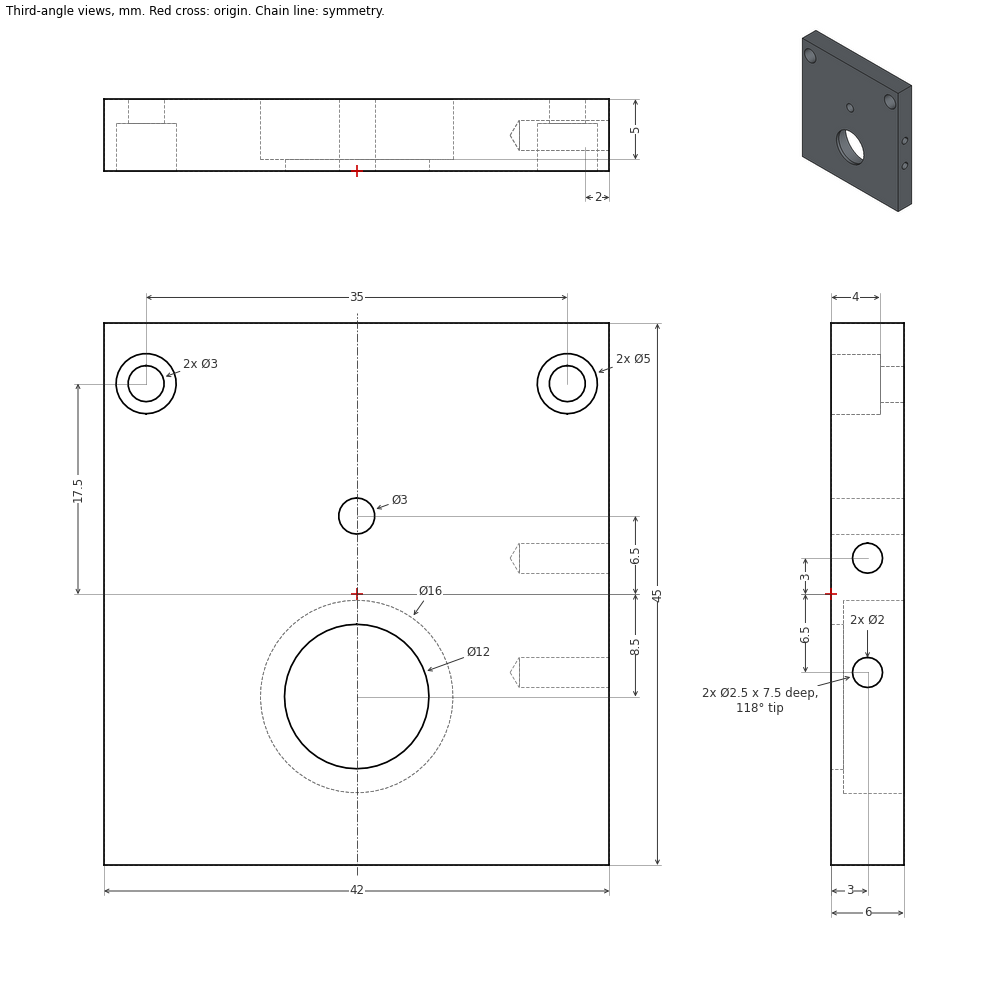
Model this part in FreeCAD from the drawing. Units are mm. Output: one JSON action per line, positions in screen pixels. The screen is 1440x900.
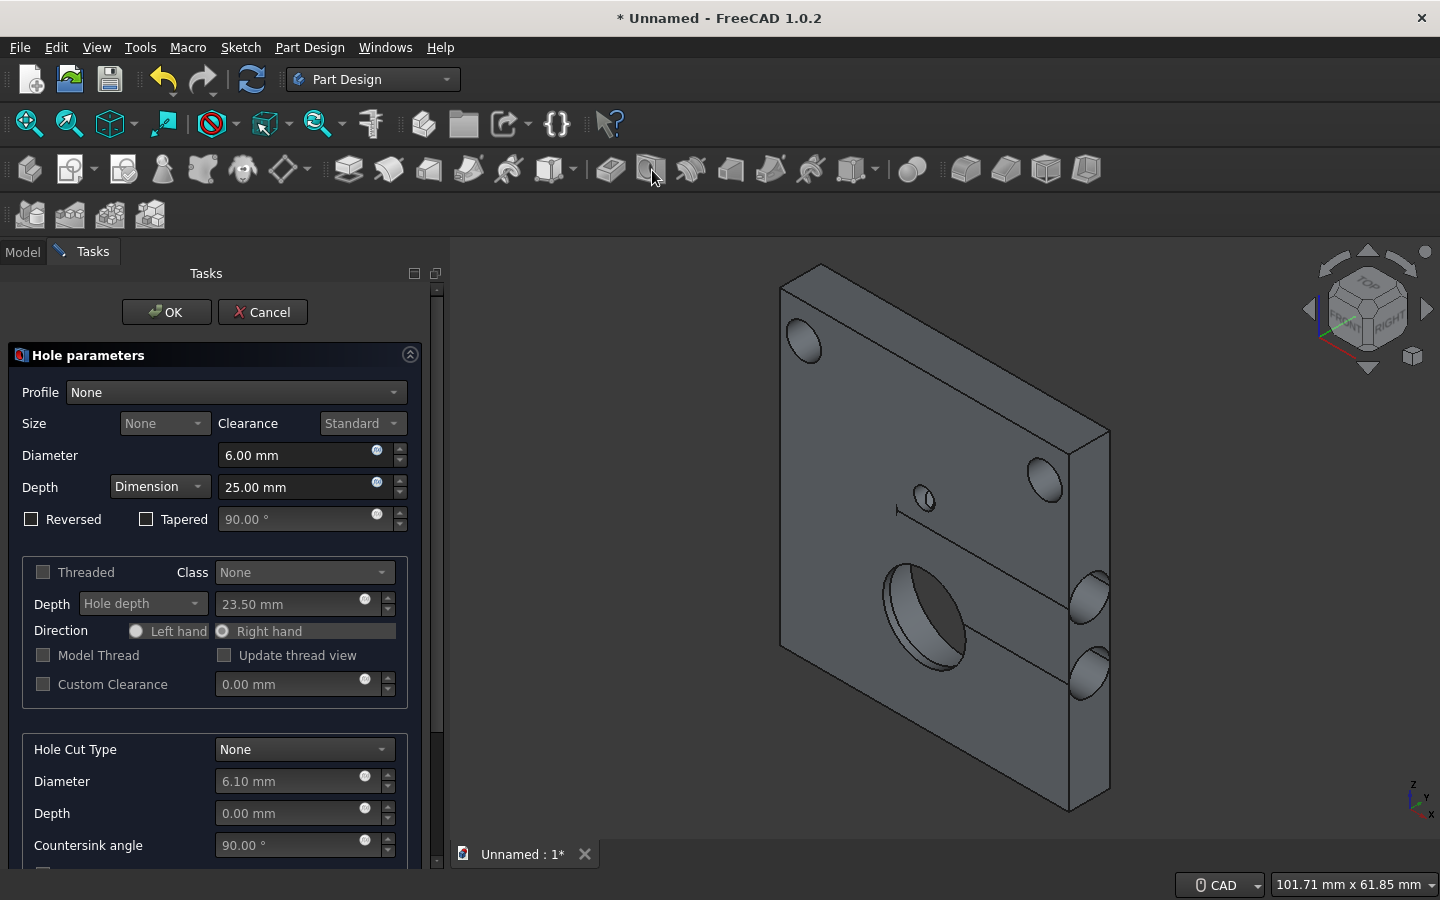
{"action": "triple_click", "coordinate": [305, 455]}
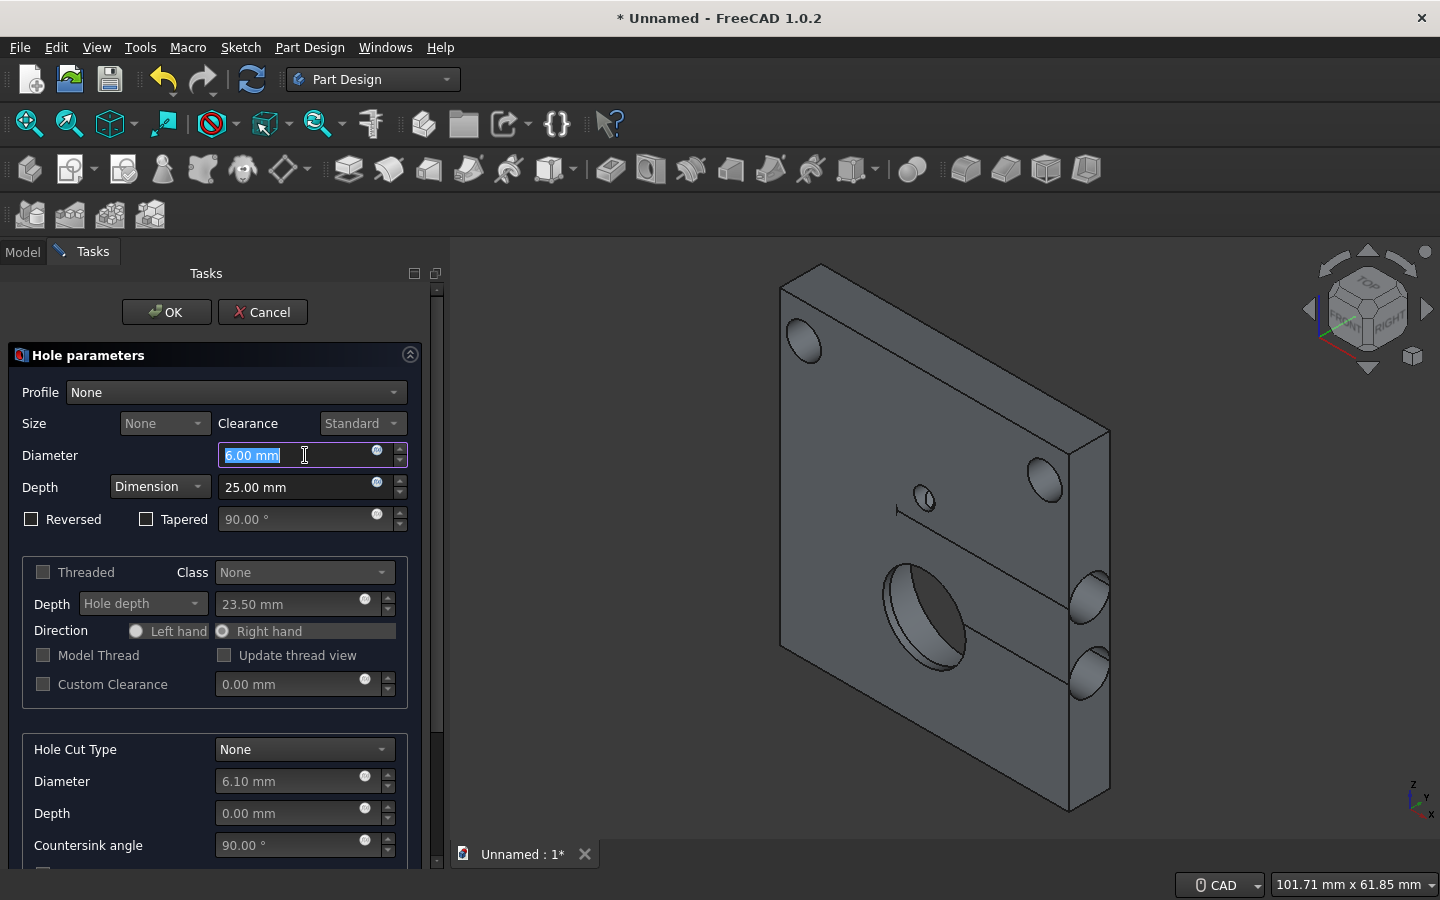
{"action": "type", "text": "2.5"}
{"action": "key", "text": "Tab"}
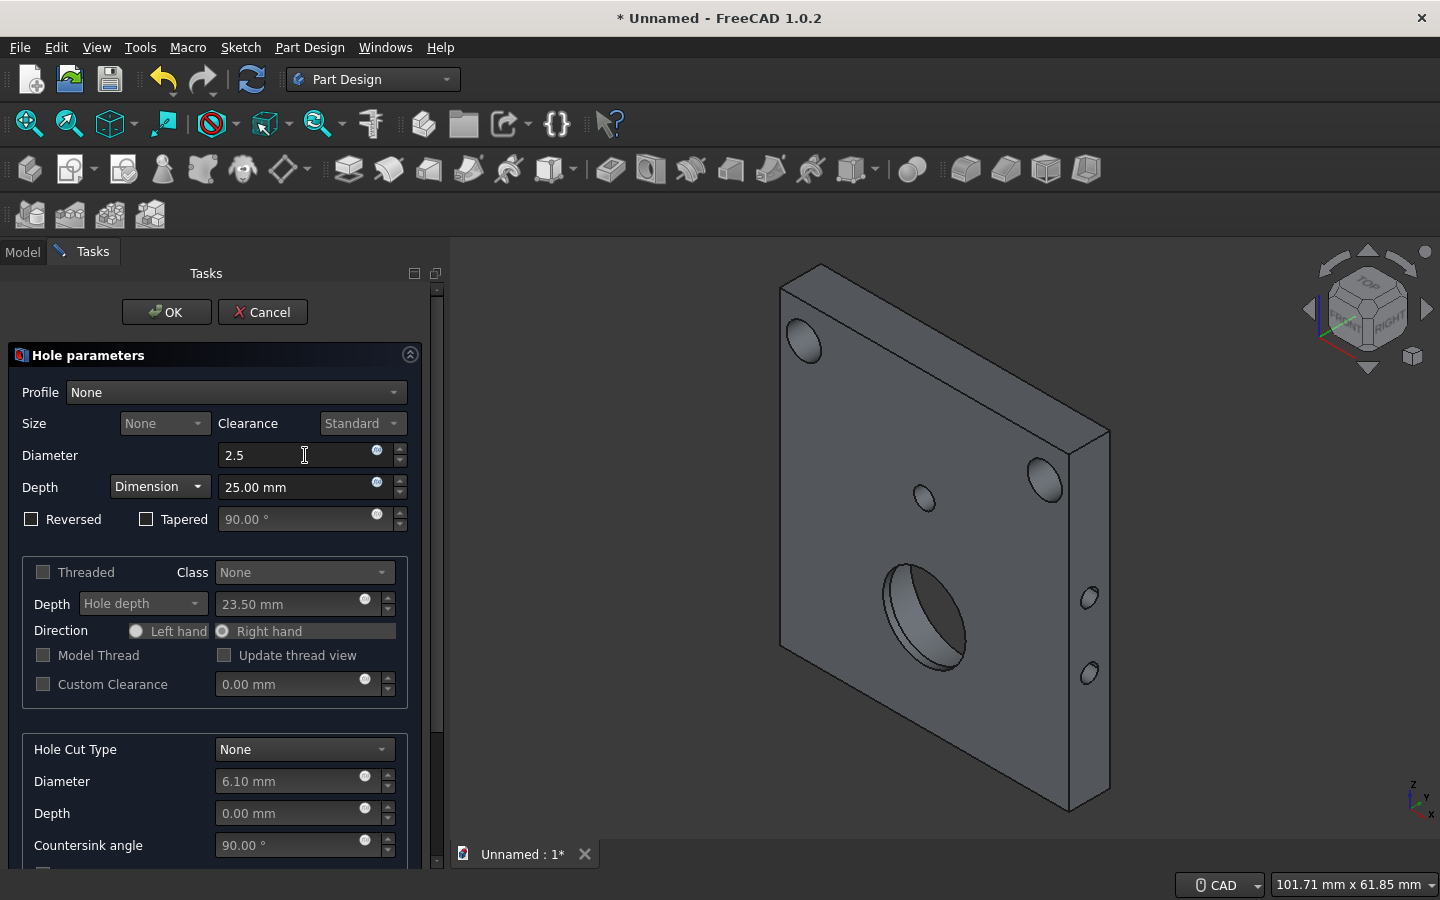
{"action": "triple_click", "coordinate": [305, 487]}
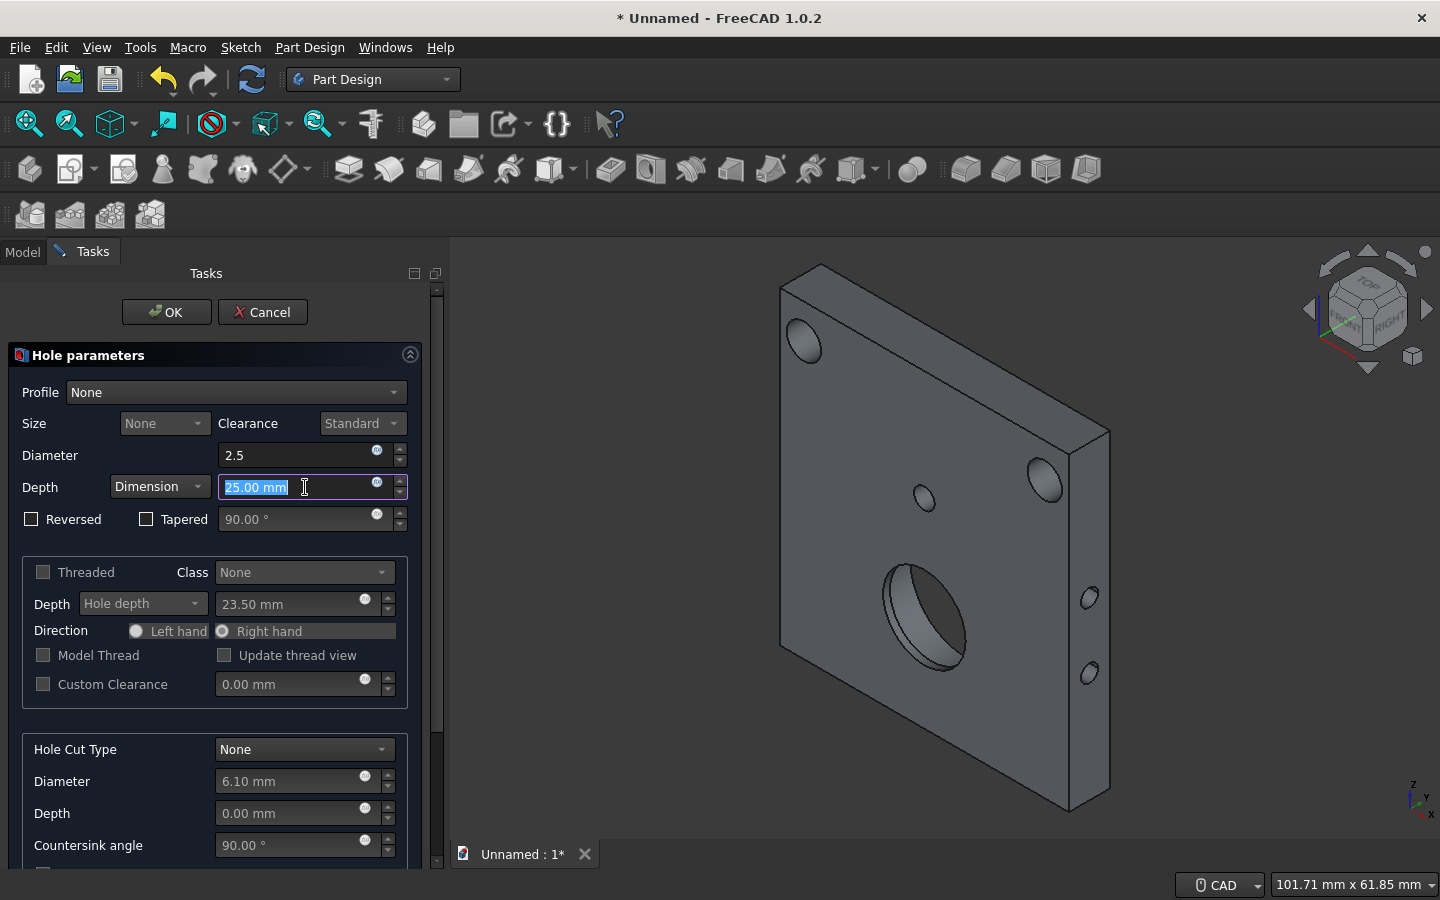
{"action": "type", "text": "7.5"}
{"action": "key", "text": "Tab"}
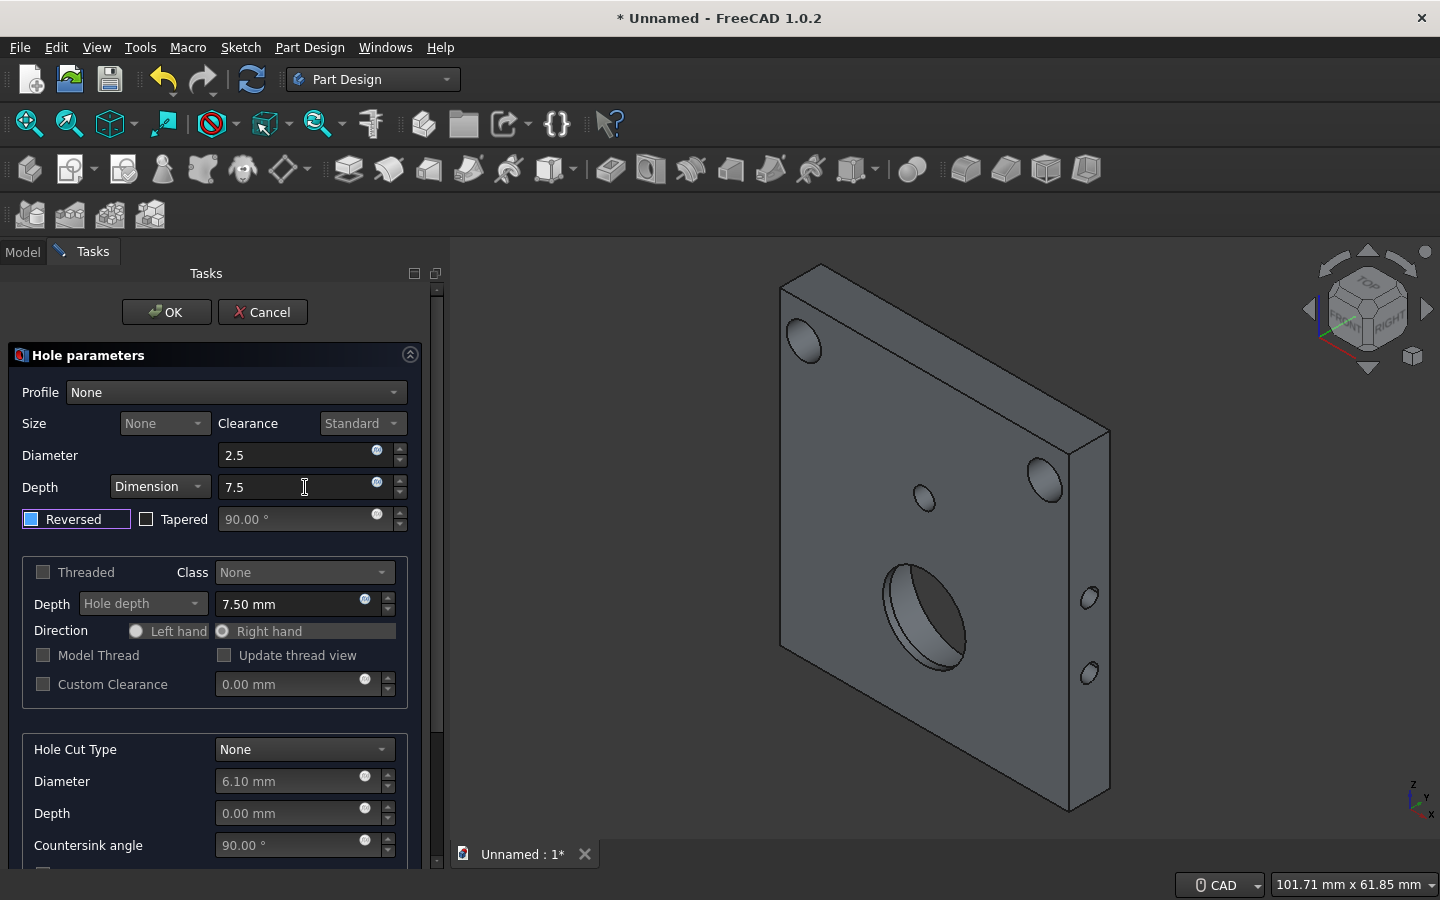
{"action": "left_click", "coordinate": [167, 312]}